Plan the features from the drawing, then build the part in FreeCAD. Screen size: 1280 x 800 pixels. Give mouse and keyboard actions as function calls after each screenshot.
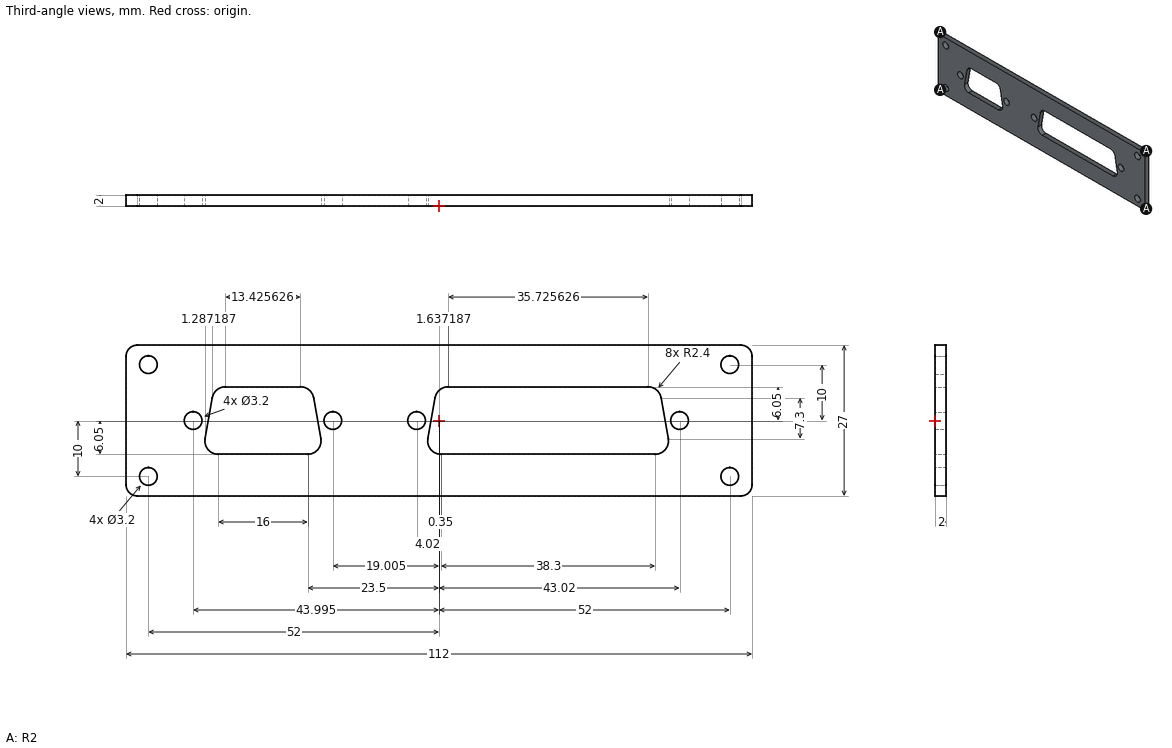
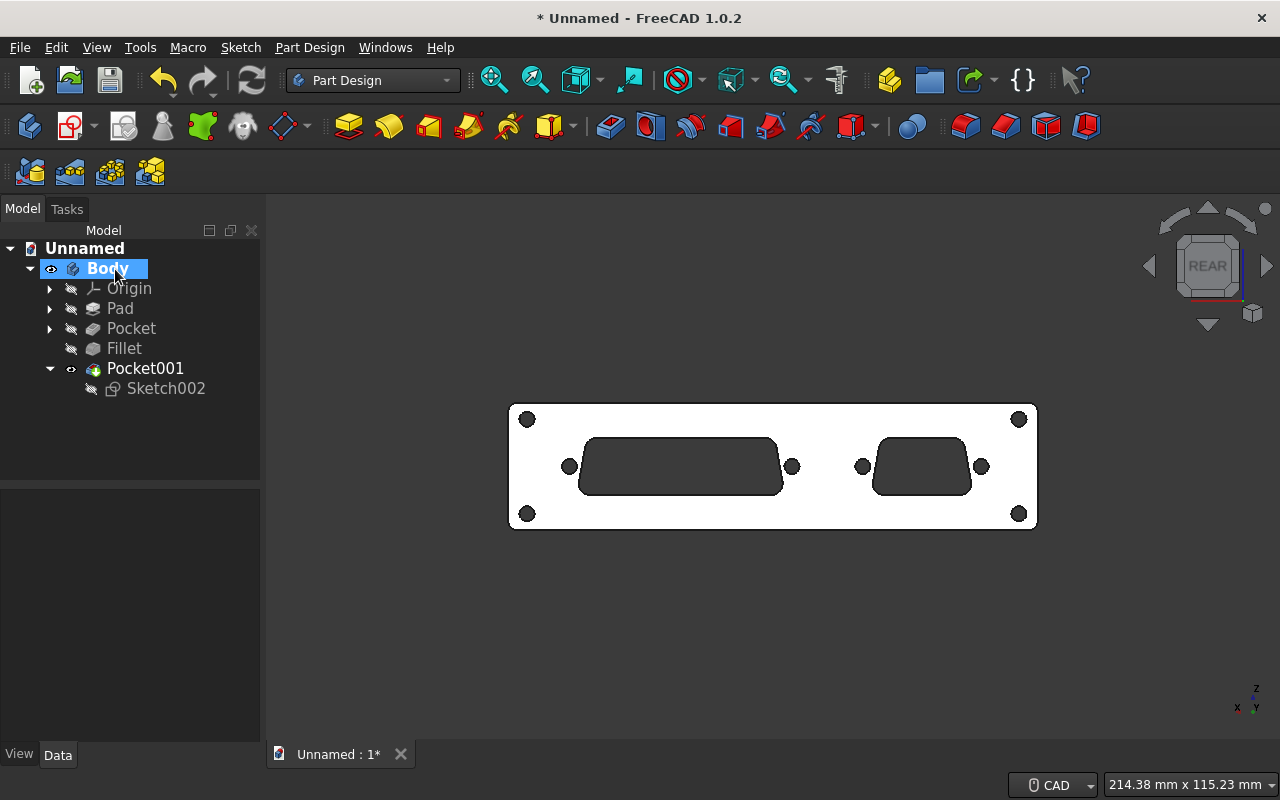
key(0)